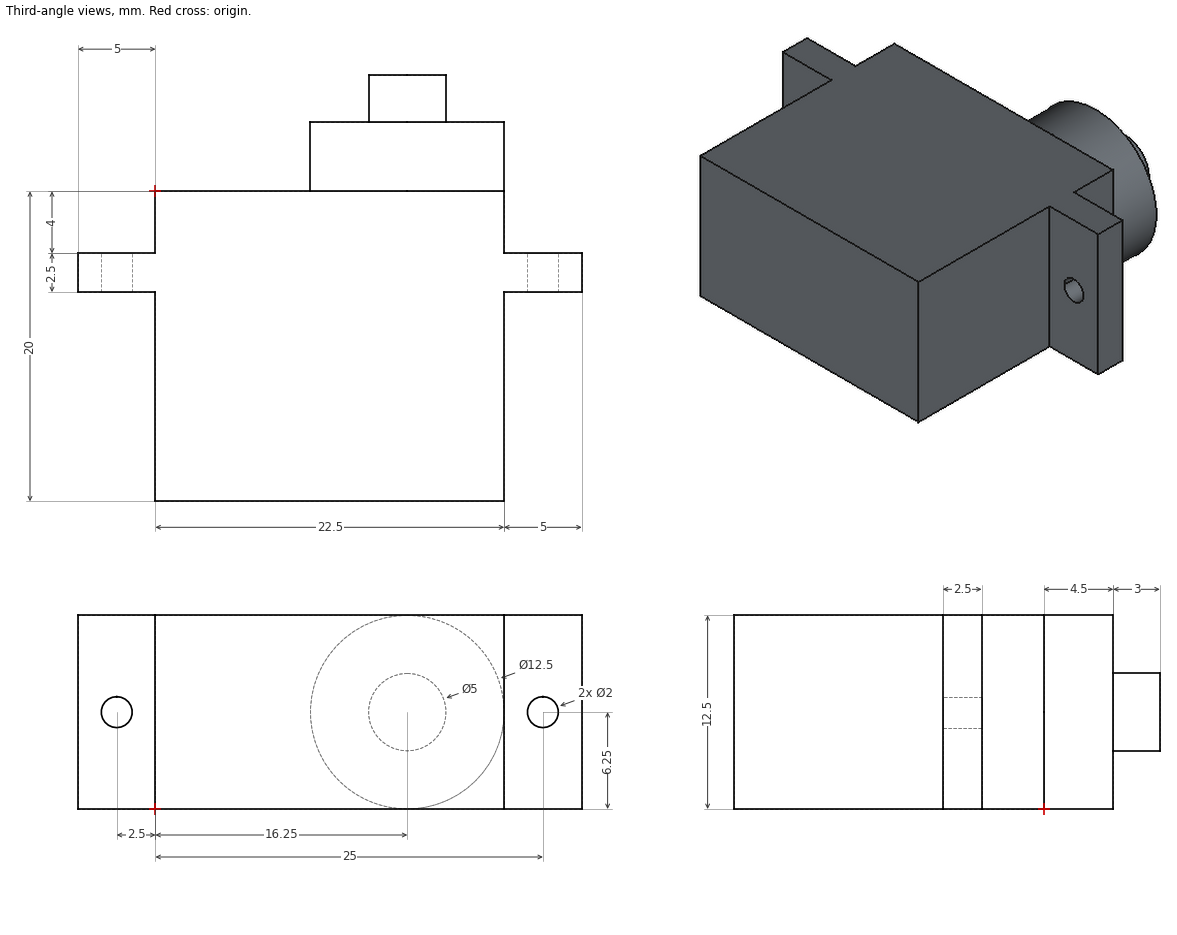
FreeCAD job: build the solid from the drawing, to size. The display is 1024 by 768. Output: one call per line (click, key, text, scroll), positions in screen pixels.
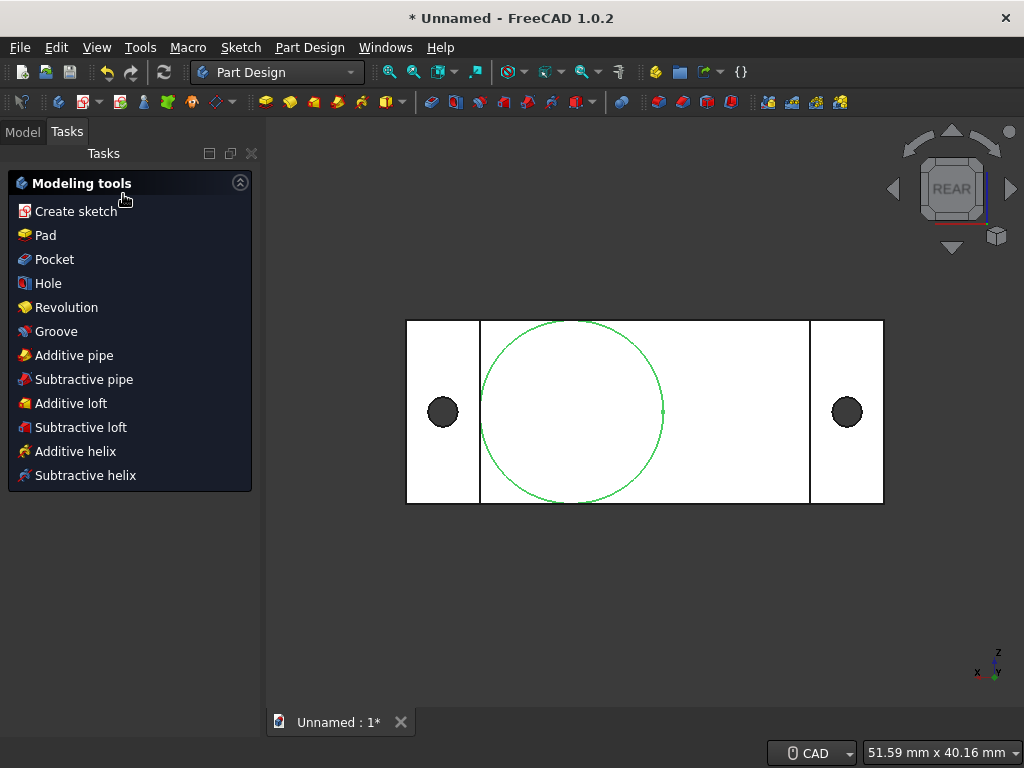
click(266, 102)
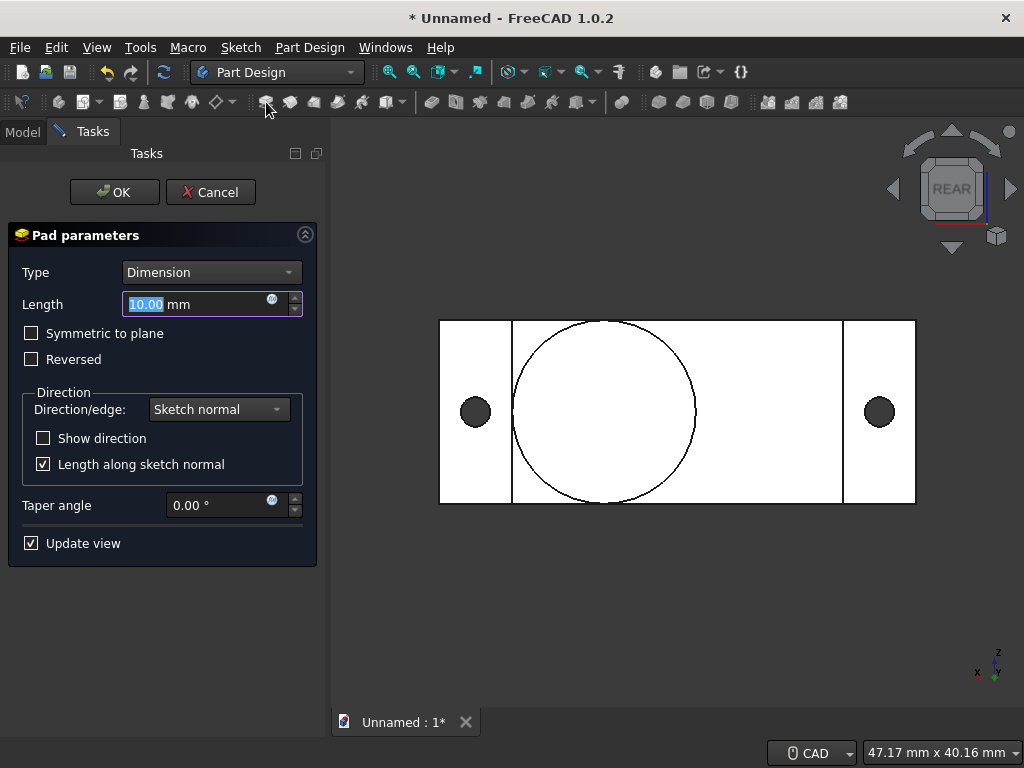
text(4.5)
key(Tab)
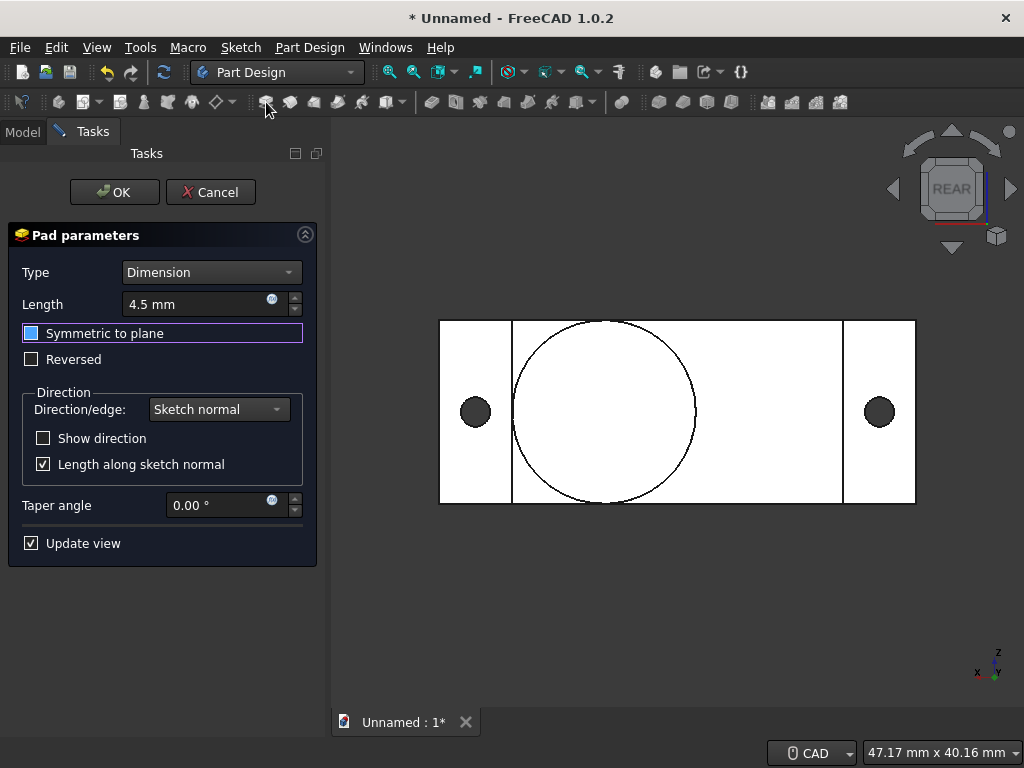
click(115, 192)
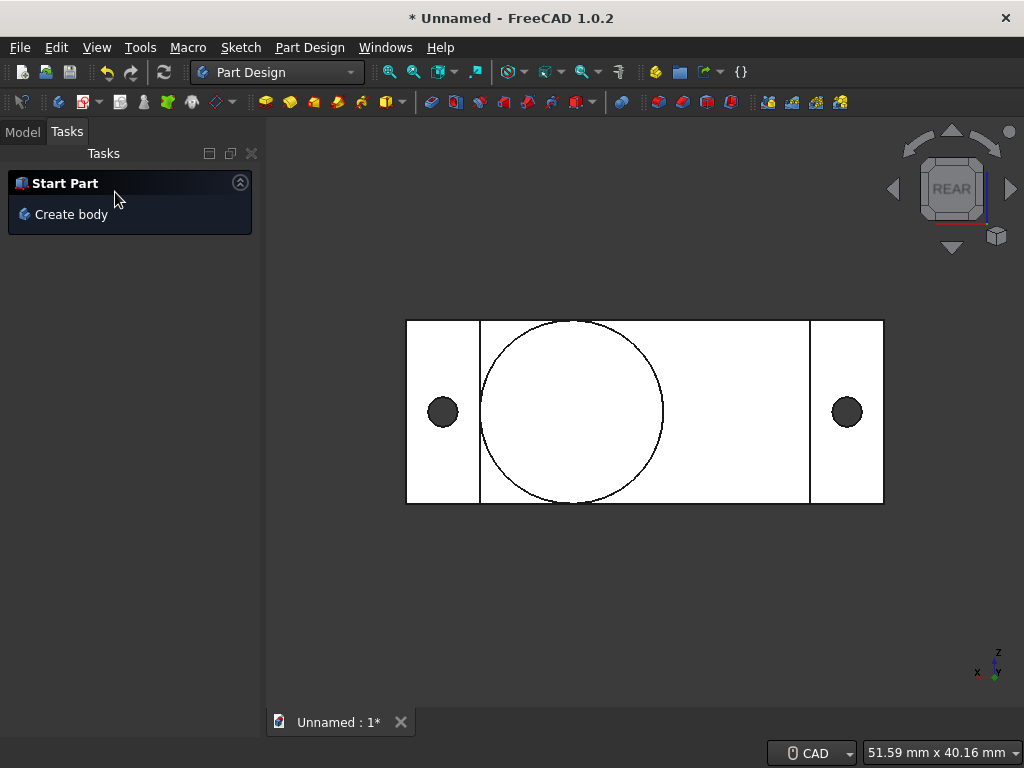
click(572, 411)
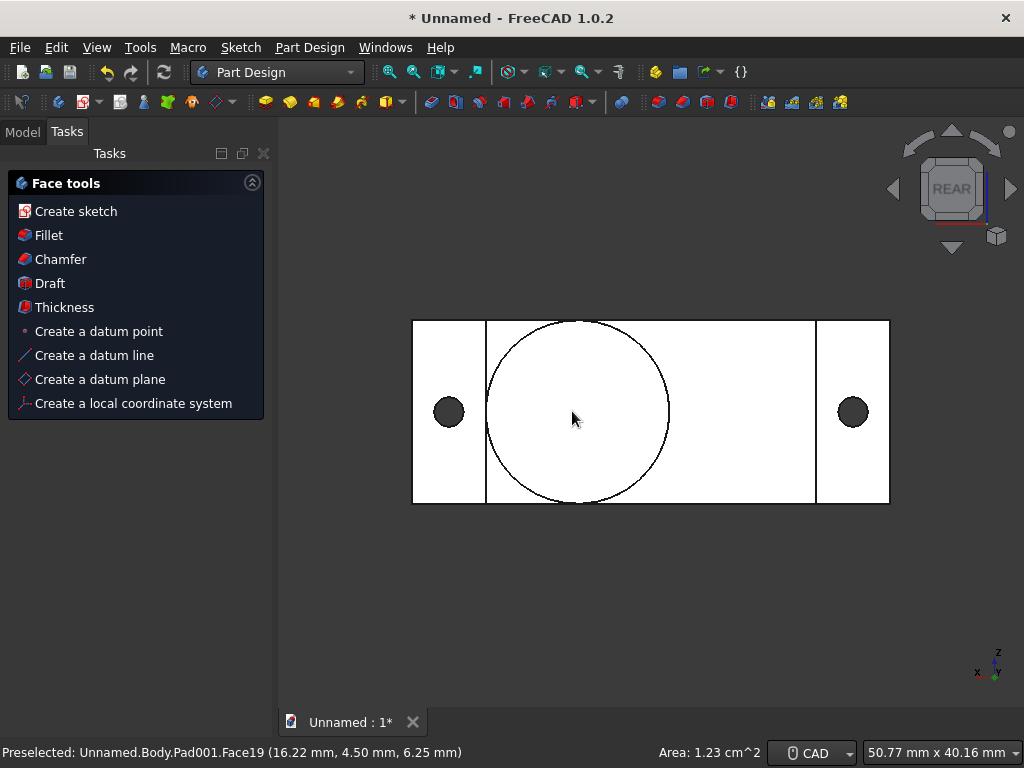
click(84, 102)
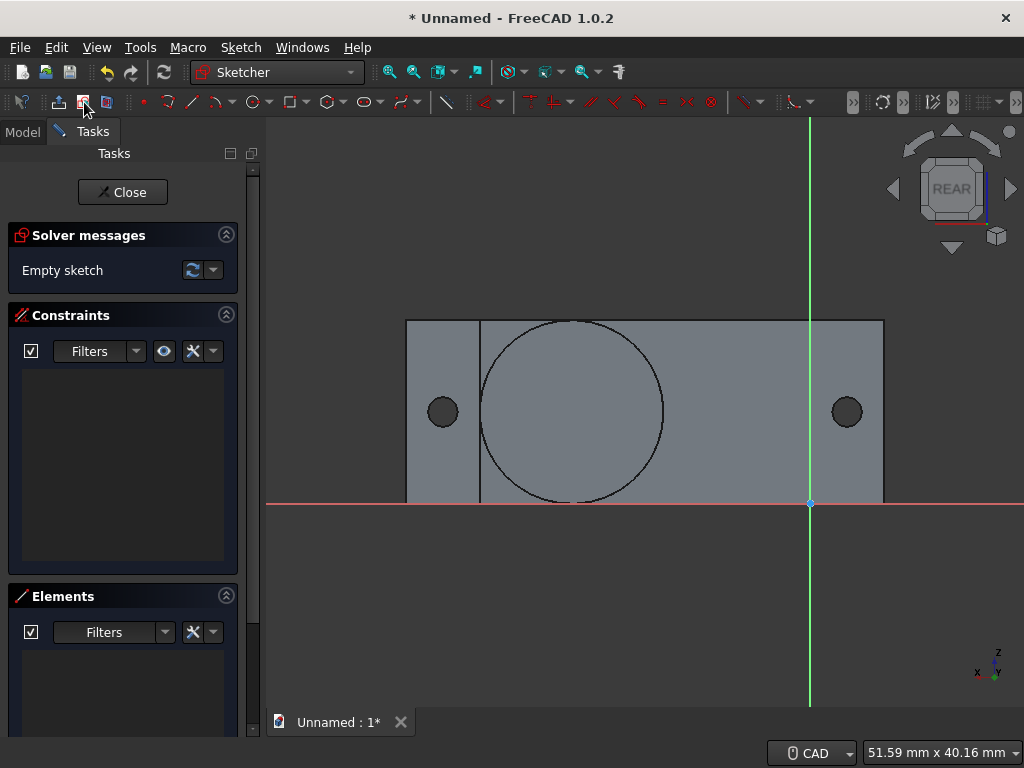
scroll(570, 412, up, 8)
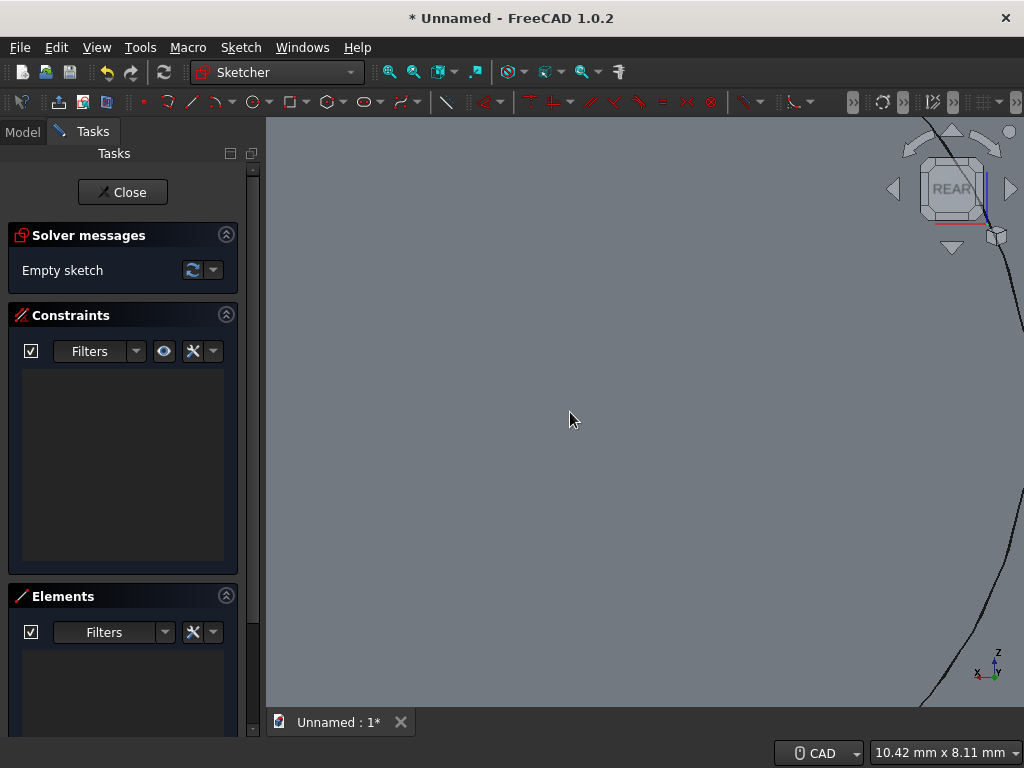
key(g)
key(c)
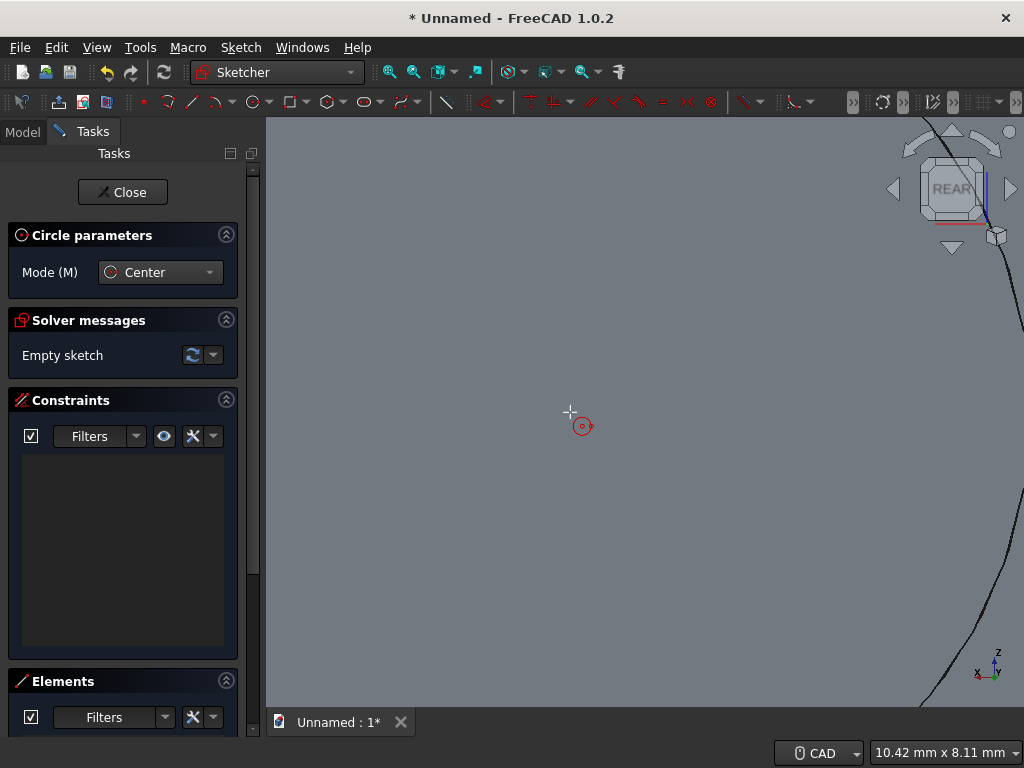
click(576, 410)
move(705, 281)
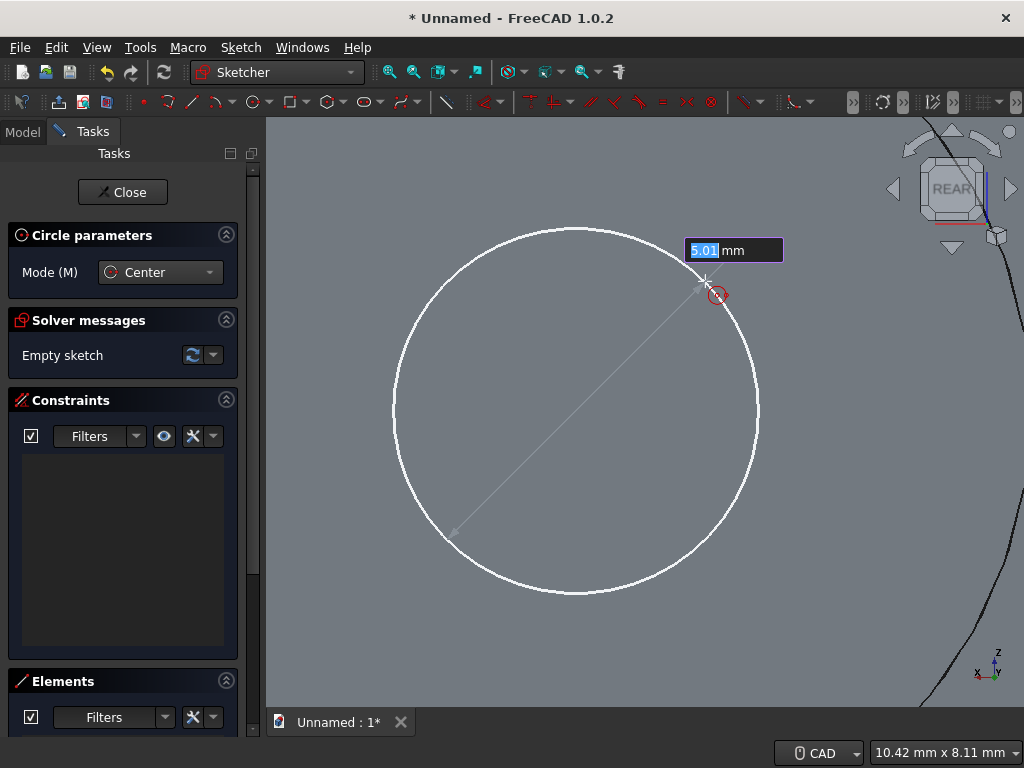
text(5)
key(Return)
key(Escape)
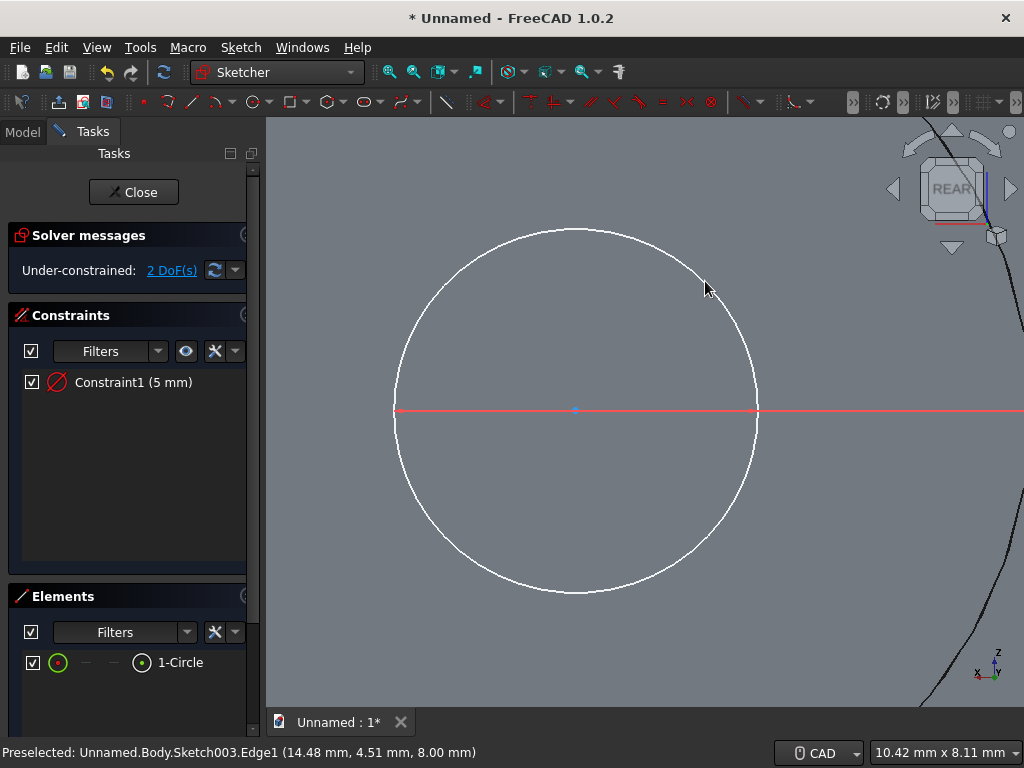
key(d)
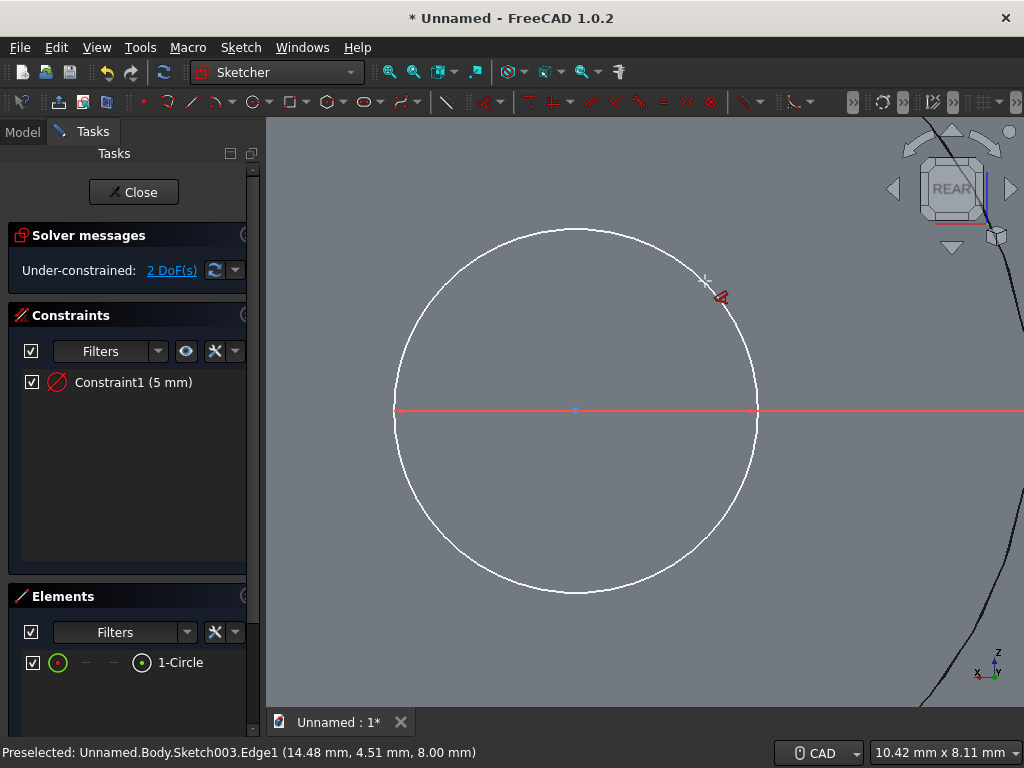
click(576, 411)
click(542, 545)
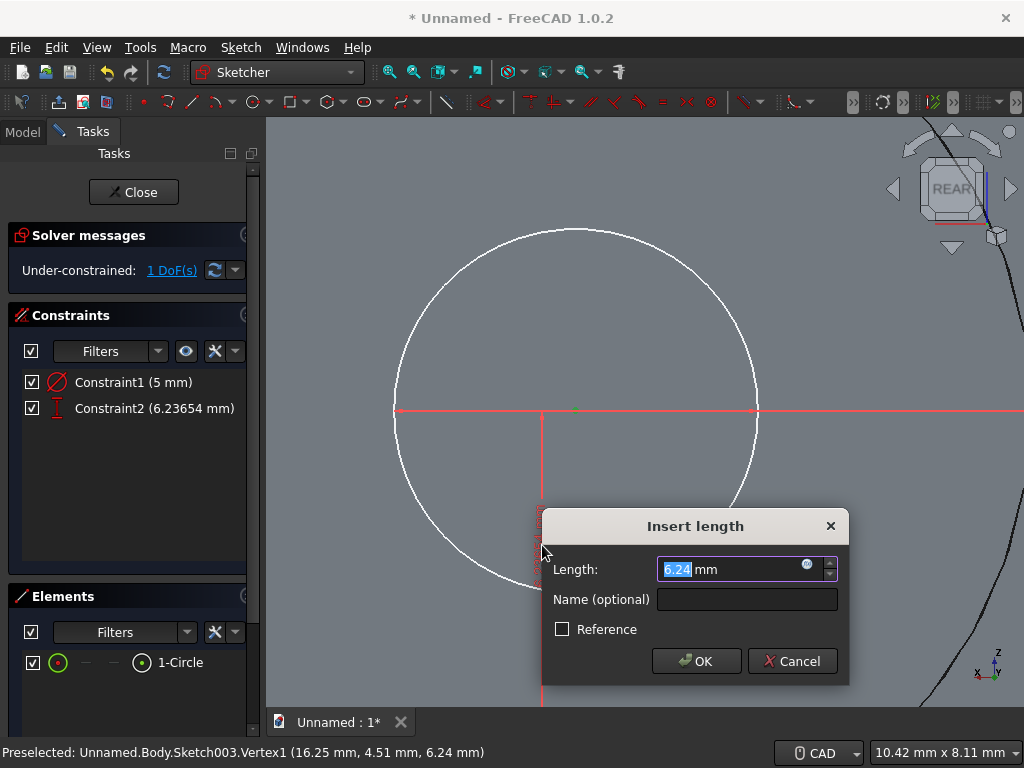
text(6.25)
key(Return)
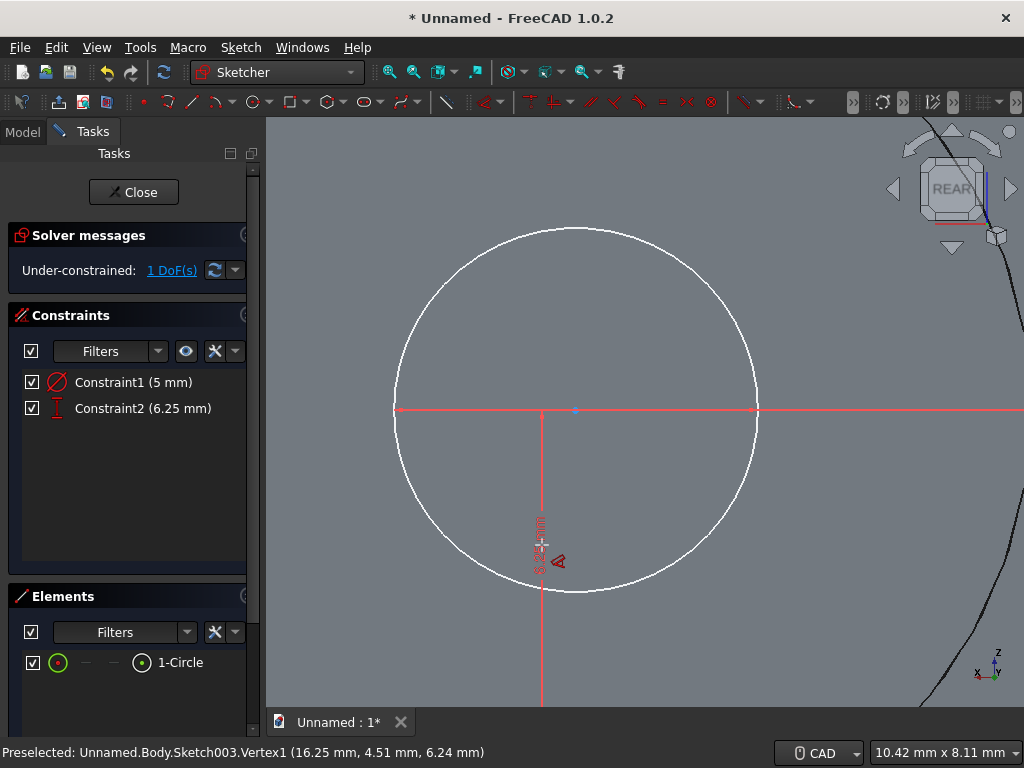
click(576, 410)
click(718, 376)